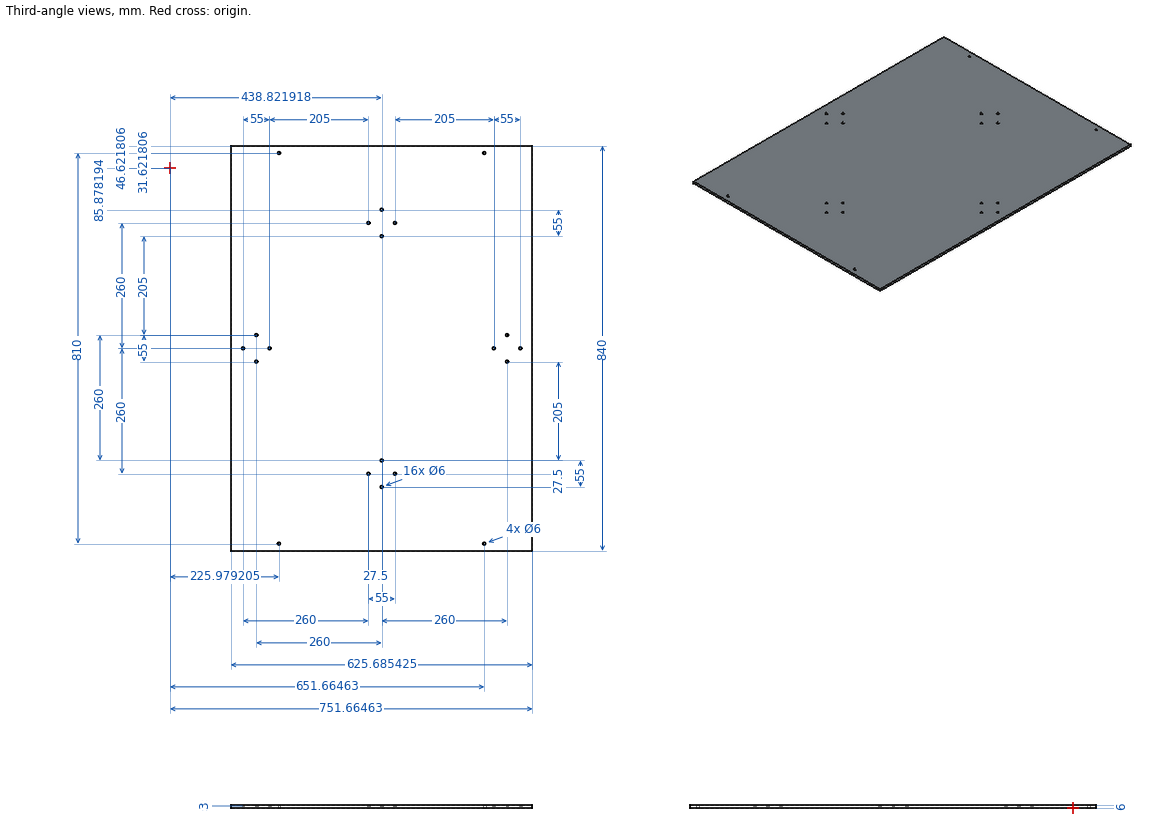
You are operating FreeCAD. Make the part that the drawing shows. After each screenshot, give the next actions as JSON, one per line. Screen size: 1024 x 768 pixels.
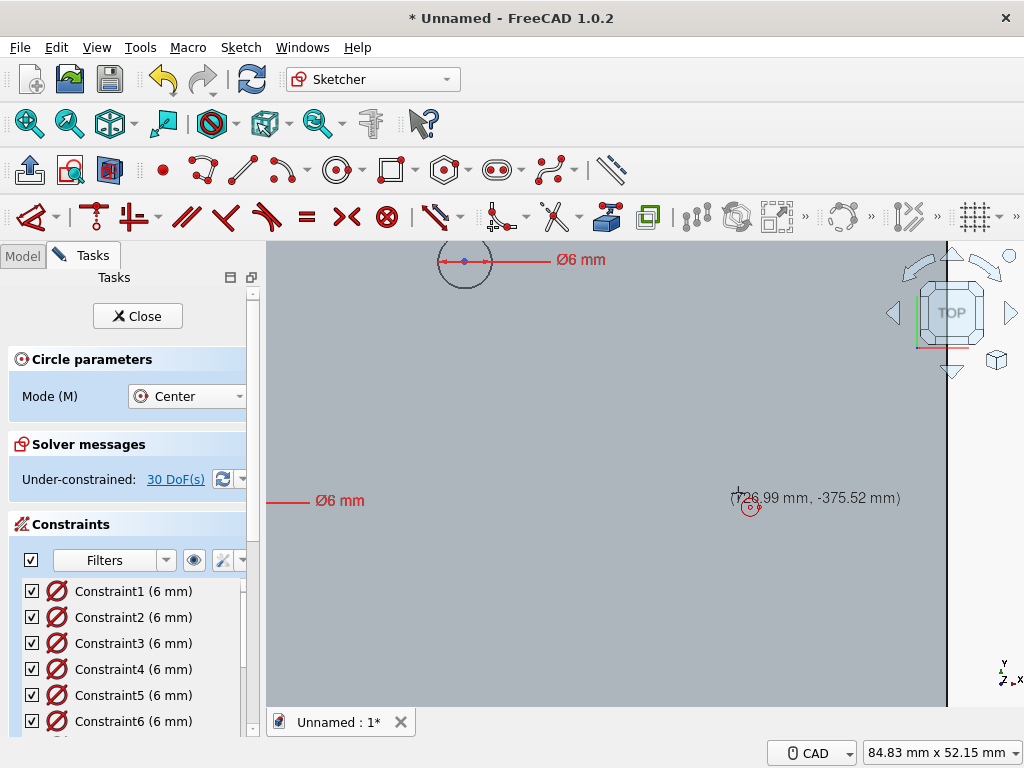
{"action": "scroll", "coordinate": [738, 493], "scroll_direction": "down", "scroll_amount": 15}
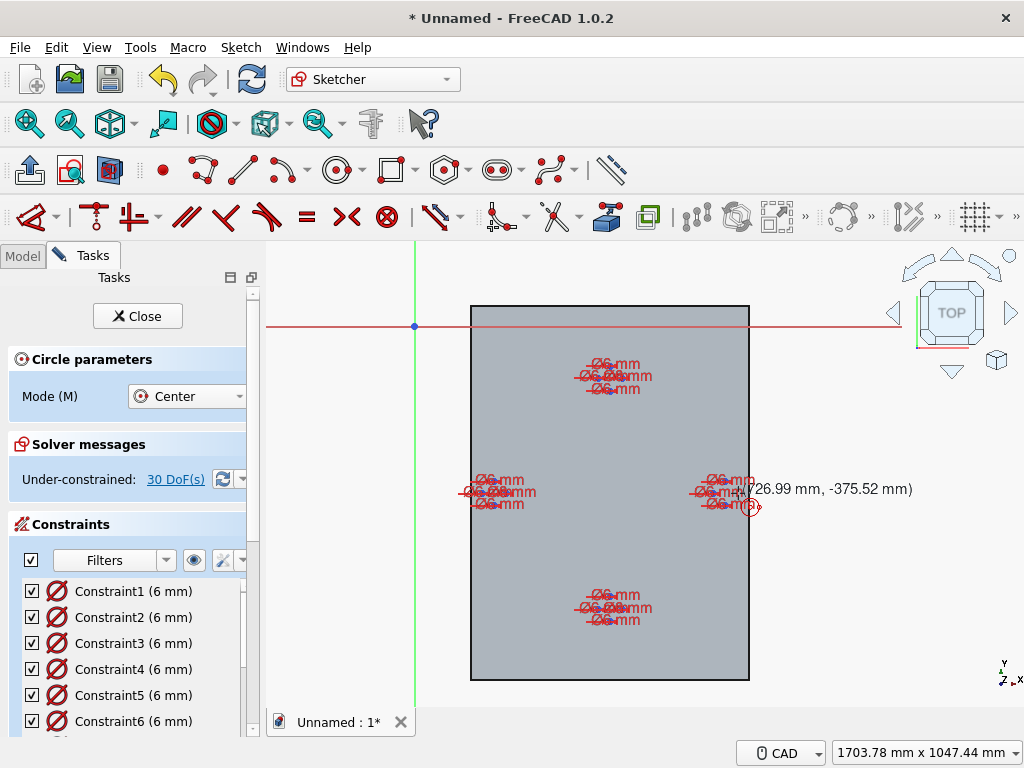
{"action": "left_click", "coordinate": [738, 493]}
{"action": "mouse_move", "coordinate": [739, 492]}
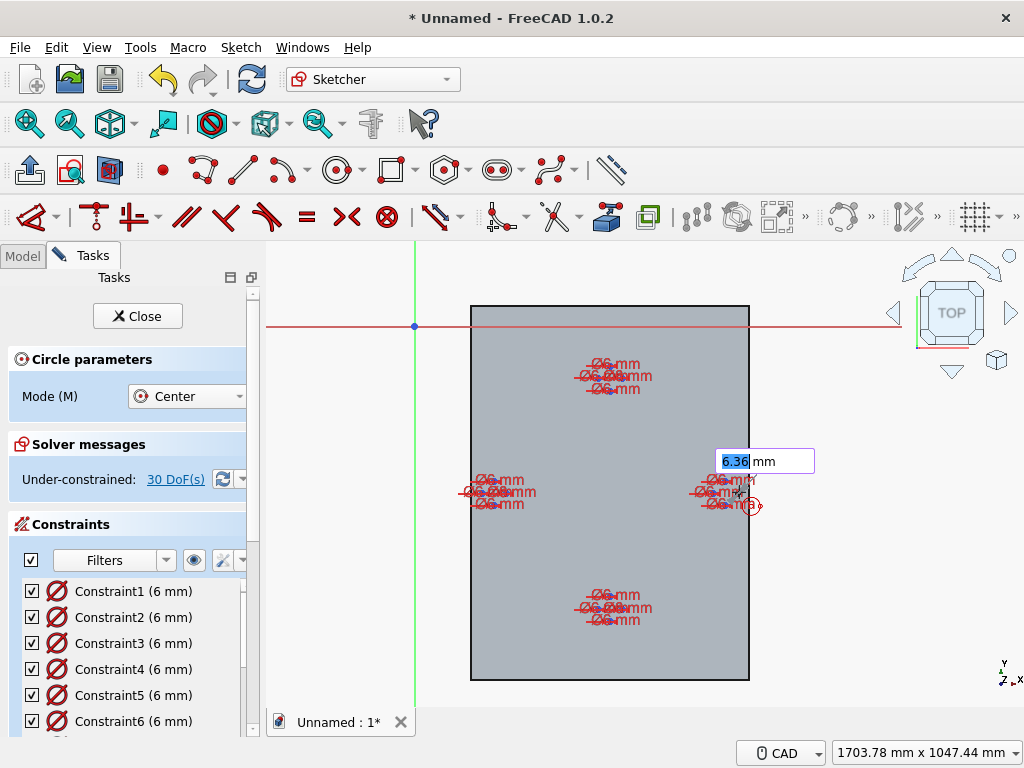
{"action": "type", "text": "6"}
{"action": "key", "text": "Return"}
{"action": "key", "text": "Escape"}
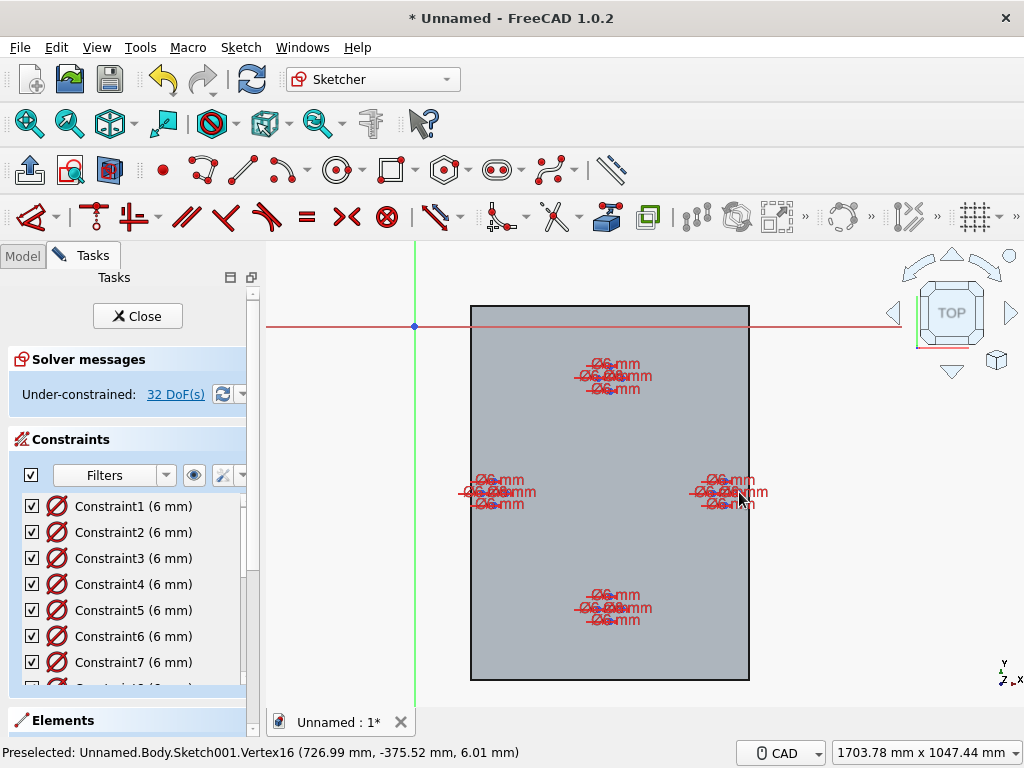
{"action": "left_click", "coordinate": [610, 622]}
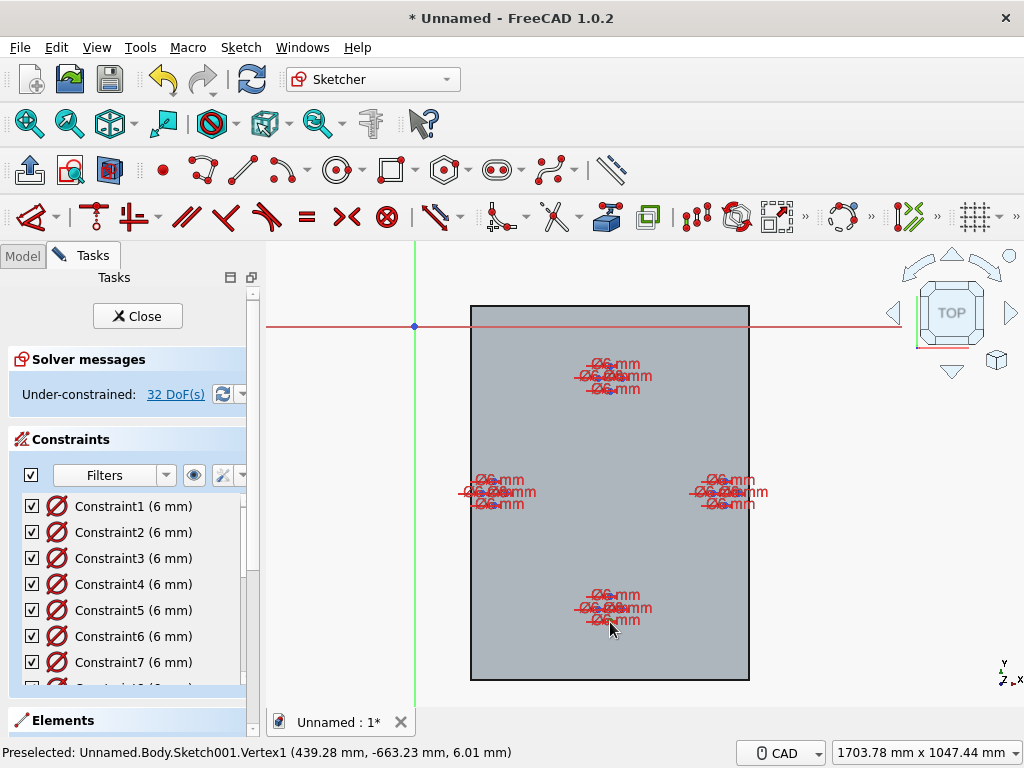
{"action": "left_click", "coordinate": [610, 597]}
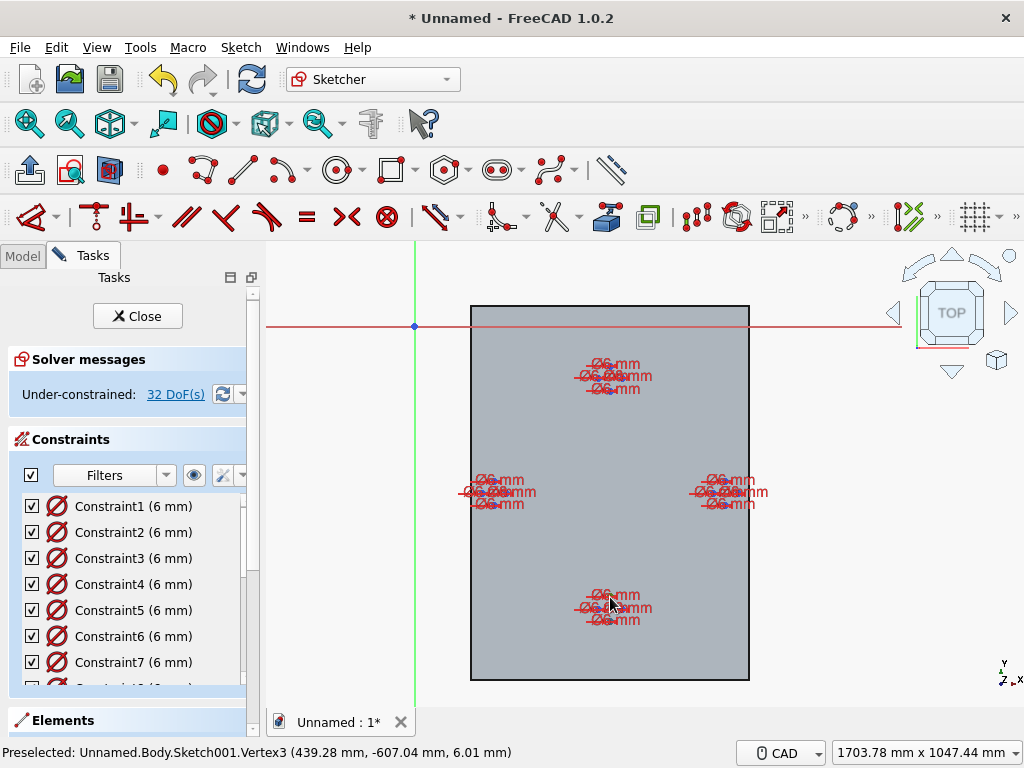
{"action": "key", "text": "v"}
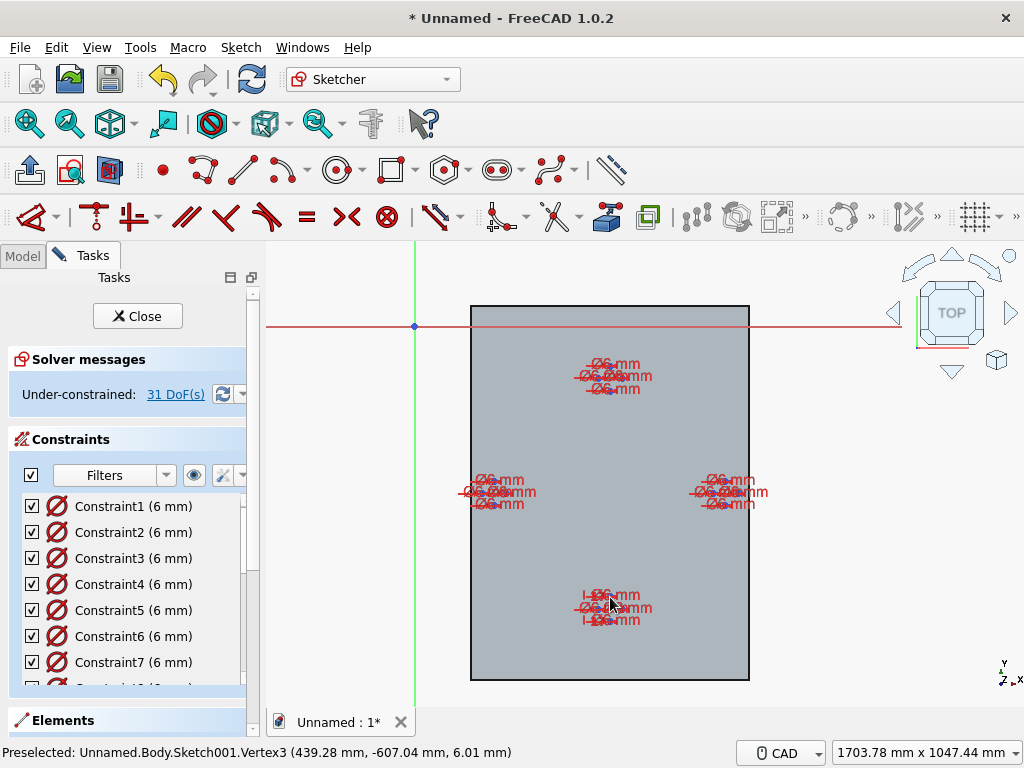
{"action": "left_click", "coordinate": [598, 610]}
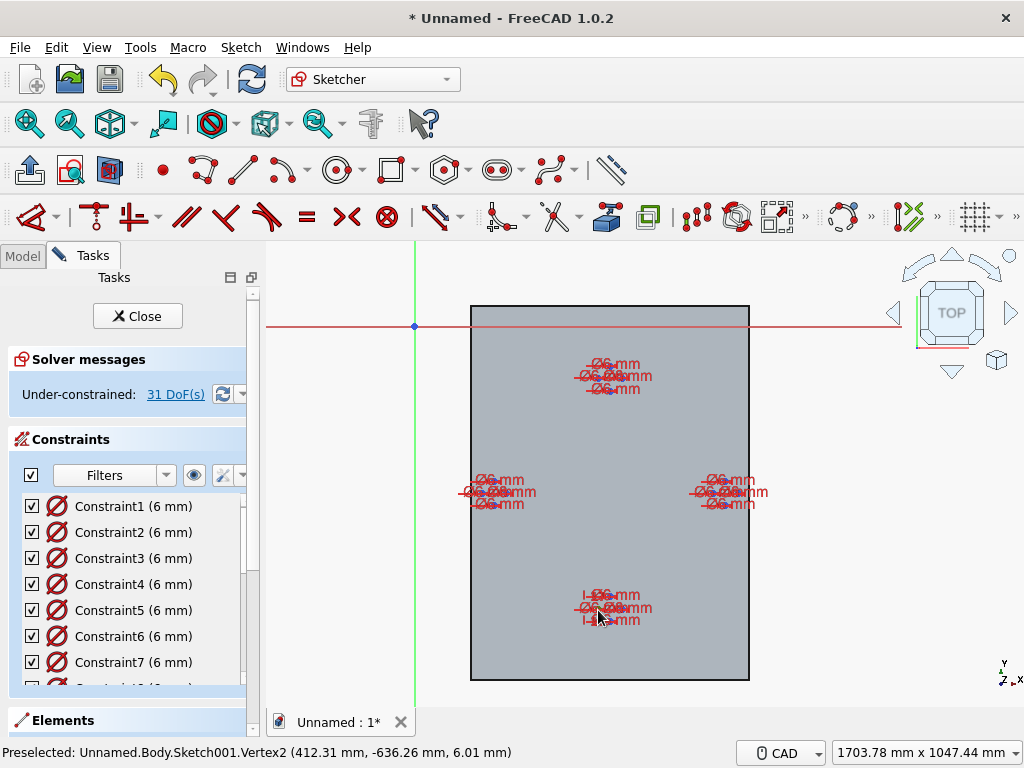
{"action": "left_click", "coordinate": [622, 610]}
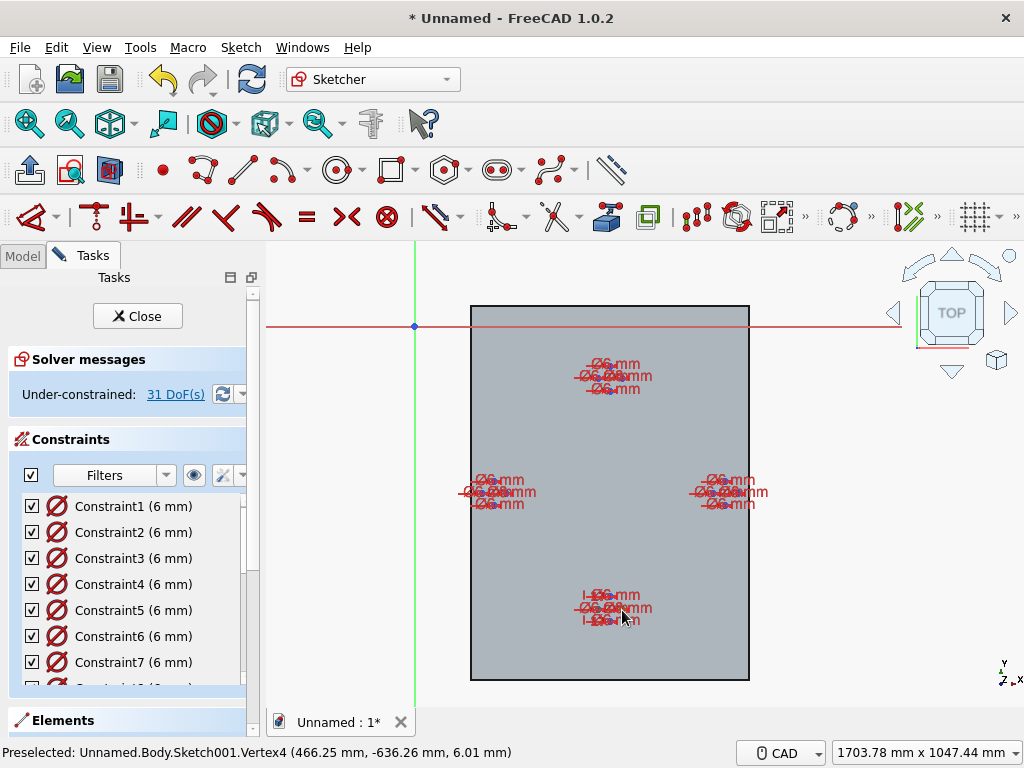
{"action": "key", "text": "h"}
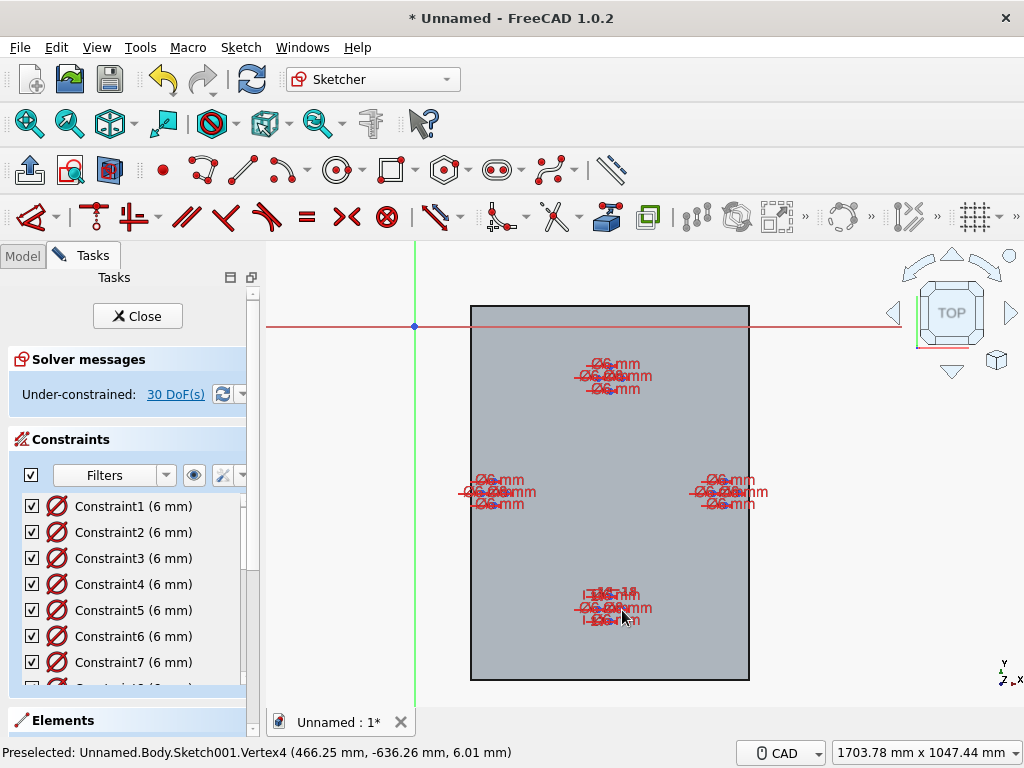
{"action": "left_click", "coordinate": [482, 494]}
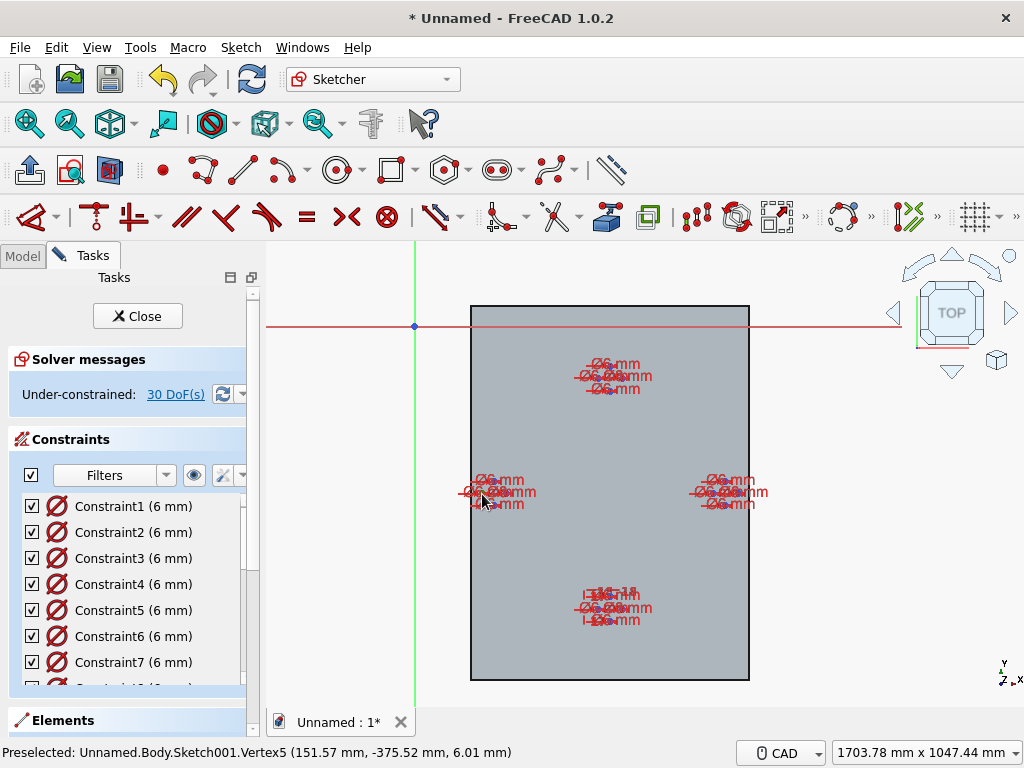
{"action": "left_click", "coordinate": [506, 494]}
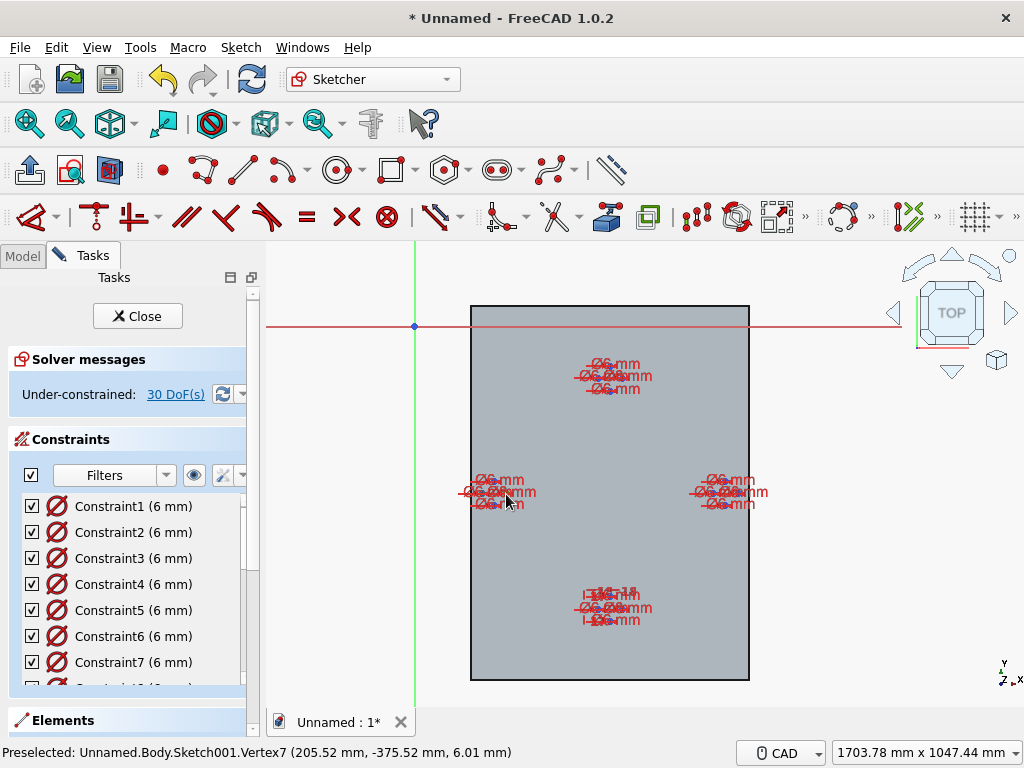
{"action": "left_click", "coordinate": [160, 218]}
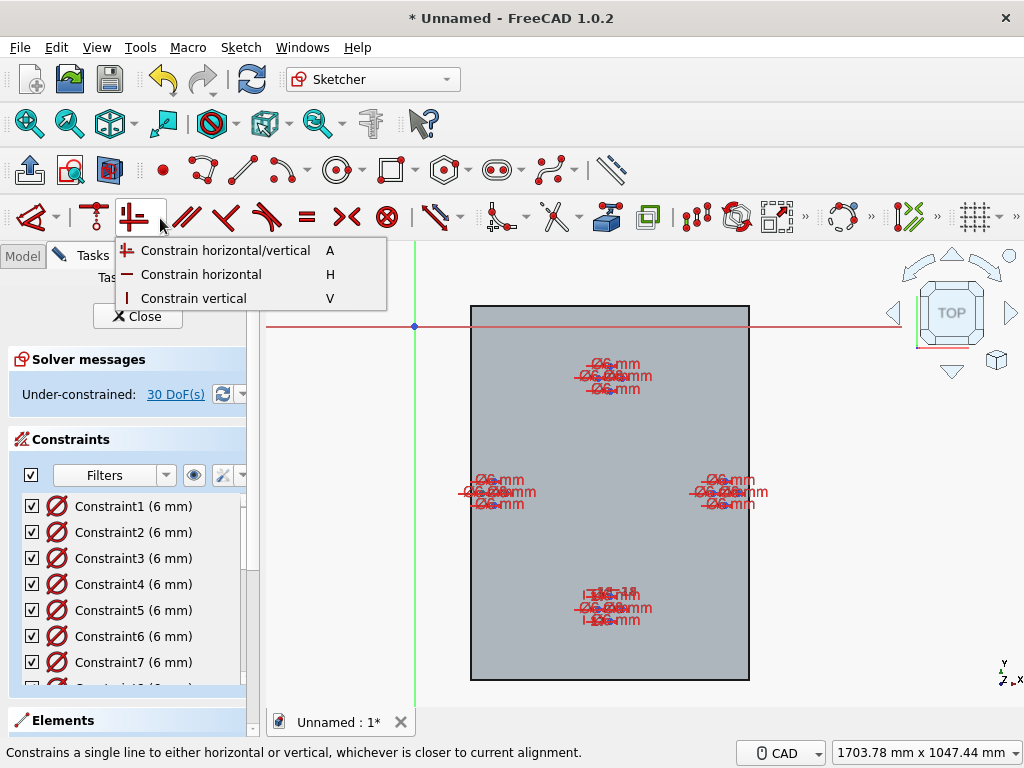
{"action": "left_click", "coordinate": [251, 274]}